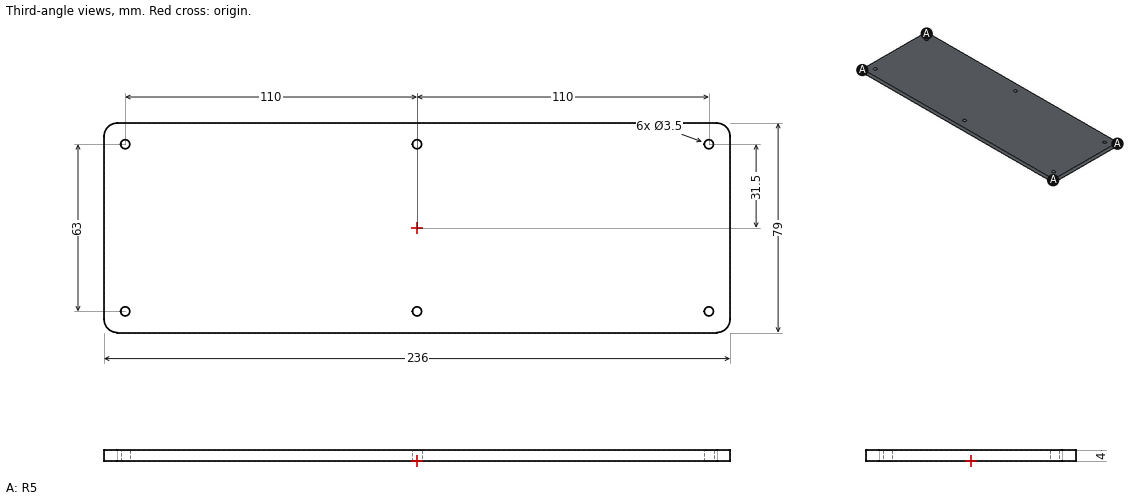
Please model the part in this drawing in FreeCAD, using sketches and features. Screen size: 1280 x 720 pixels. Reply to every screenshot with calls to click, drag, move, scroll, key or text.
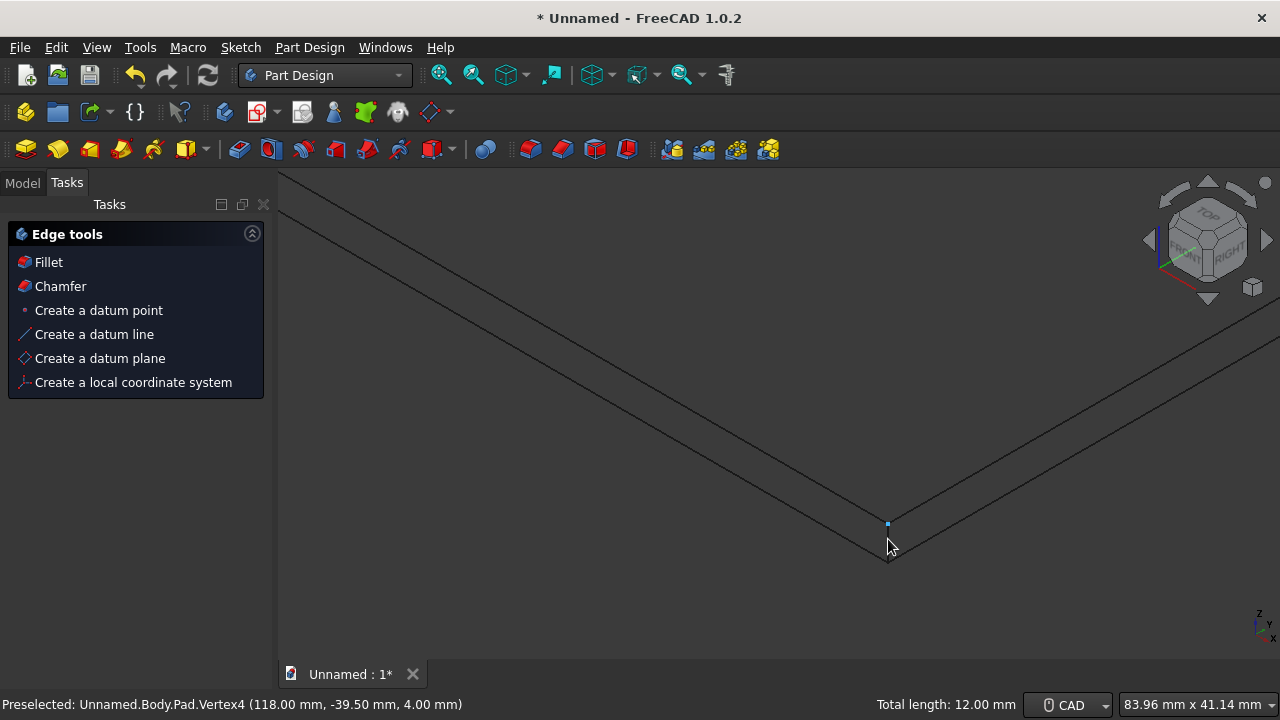
click(888, 542, ctrl)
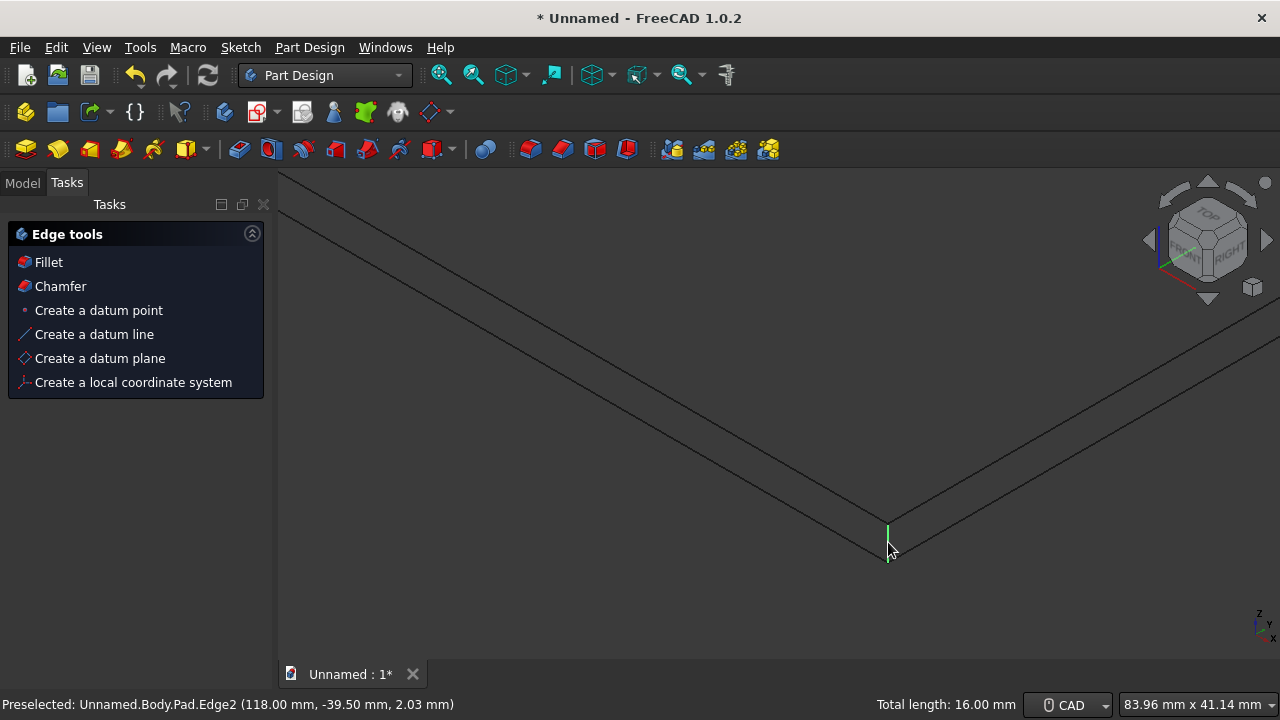
key(v)
key(1)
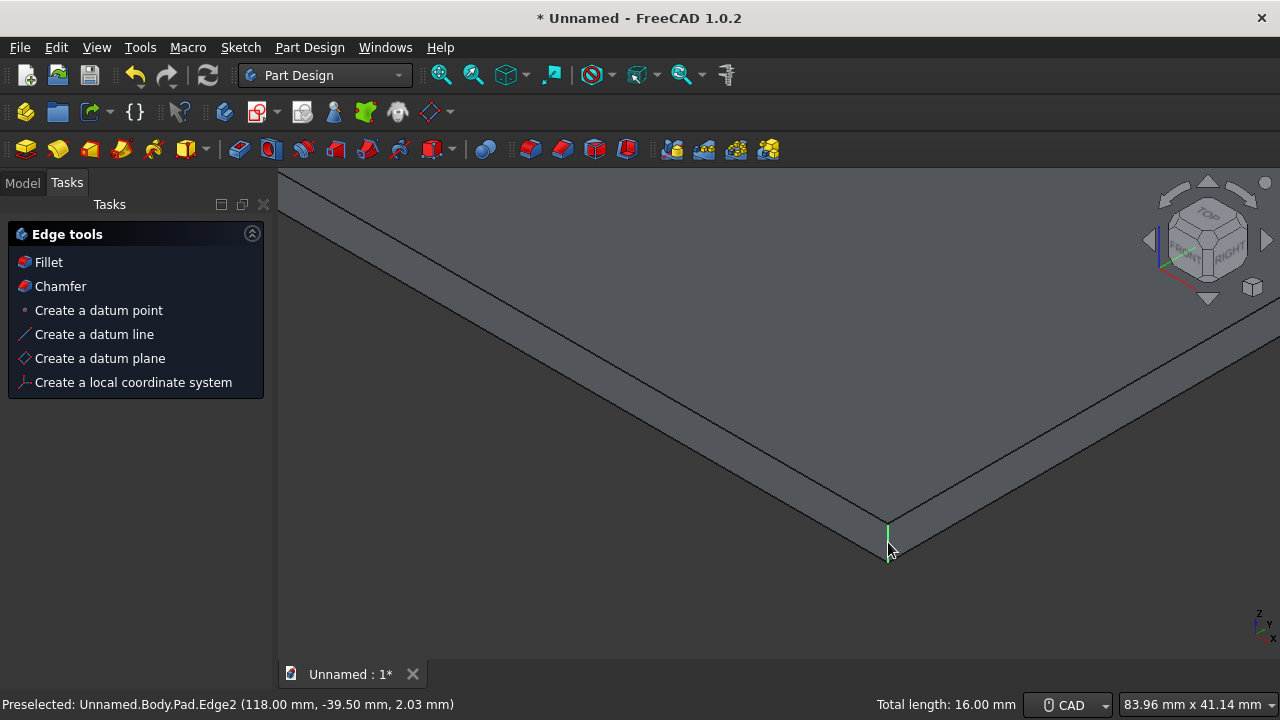
click(532, 150)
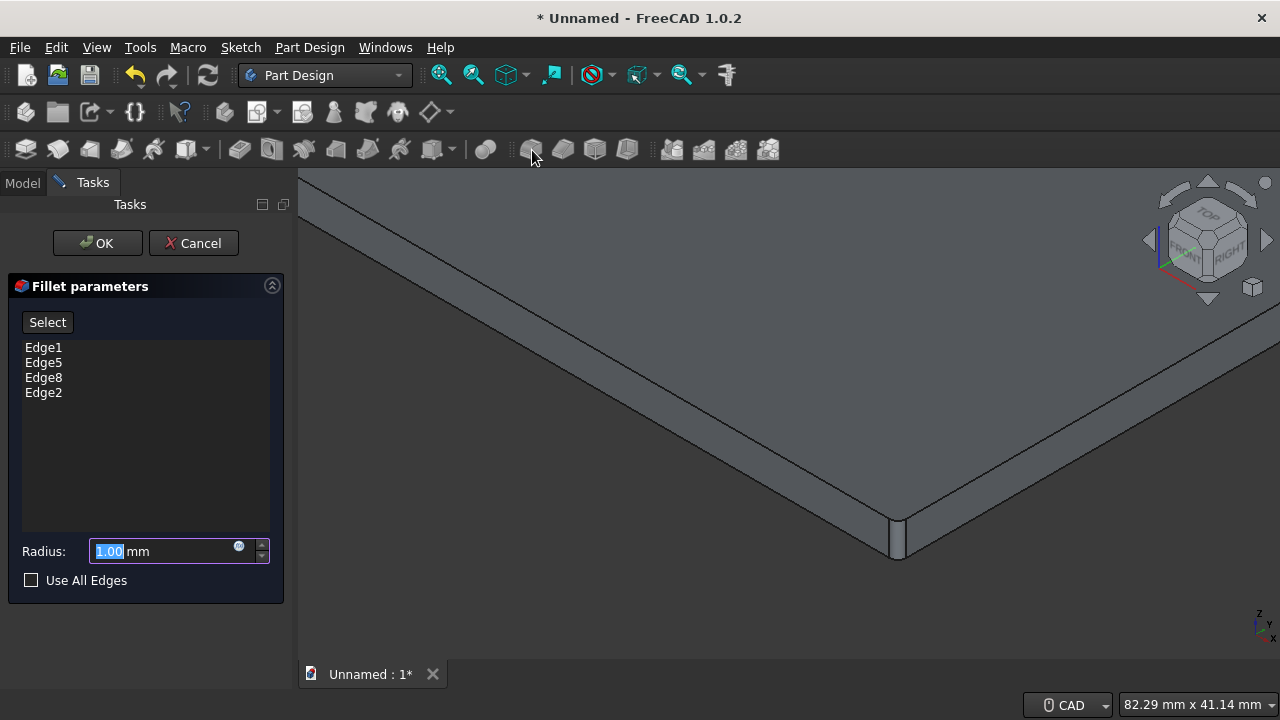
text(5)
key(Tab)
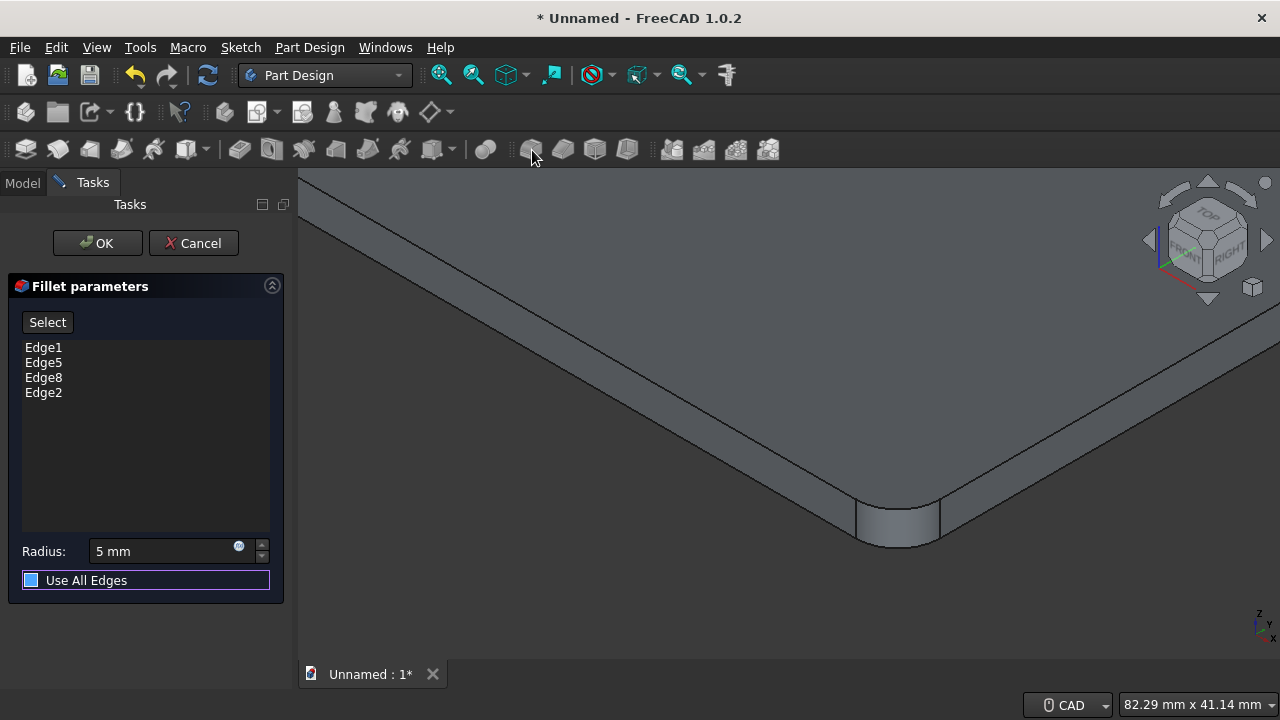
click(98, 243)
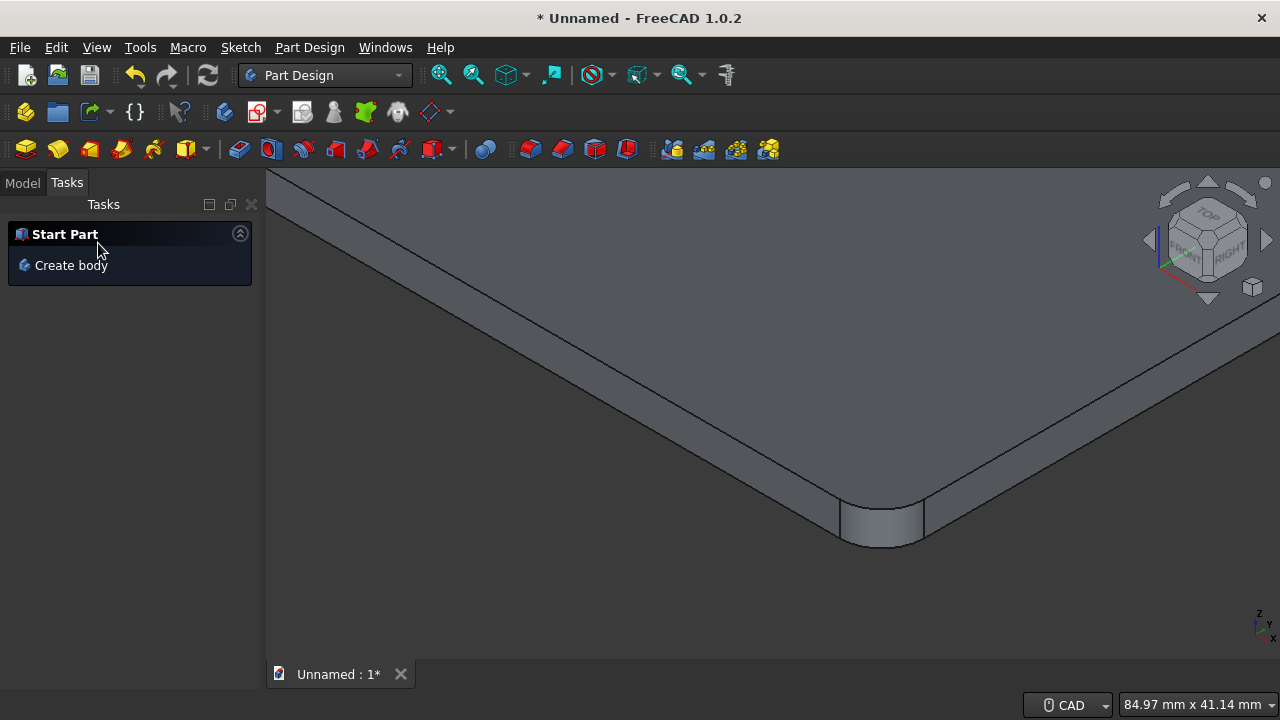
click(442, 76)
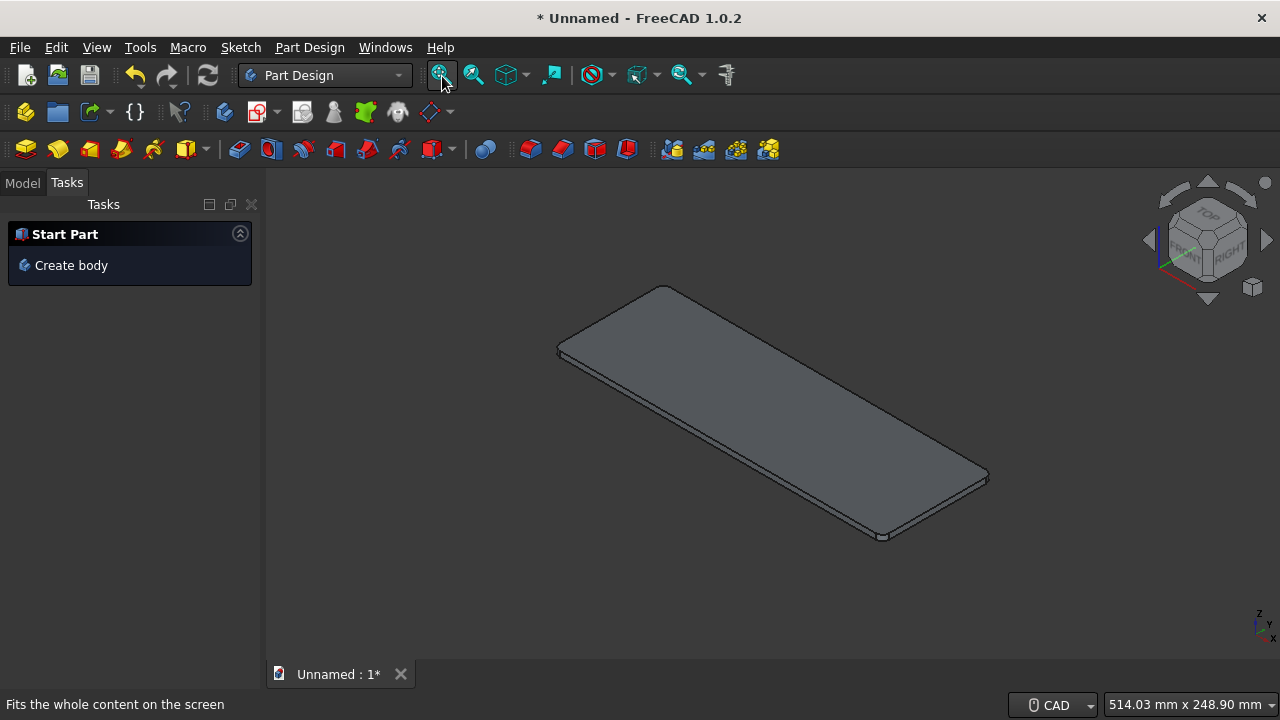
click(258, 112)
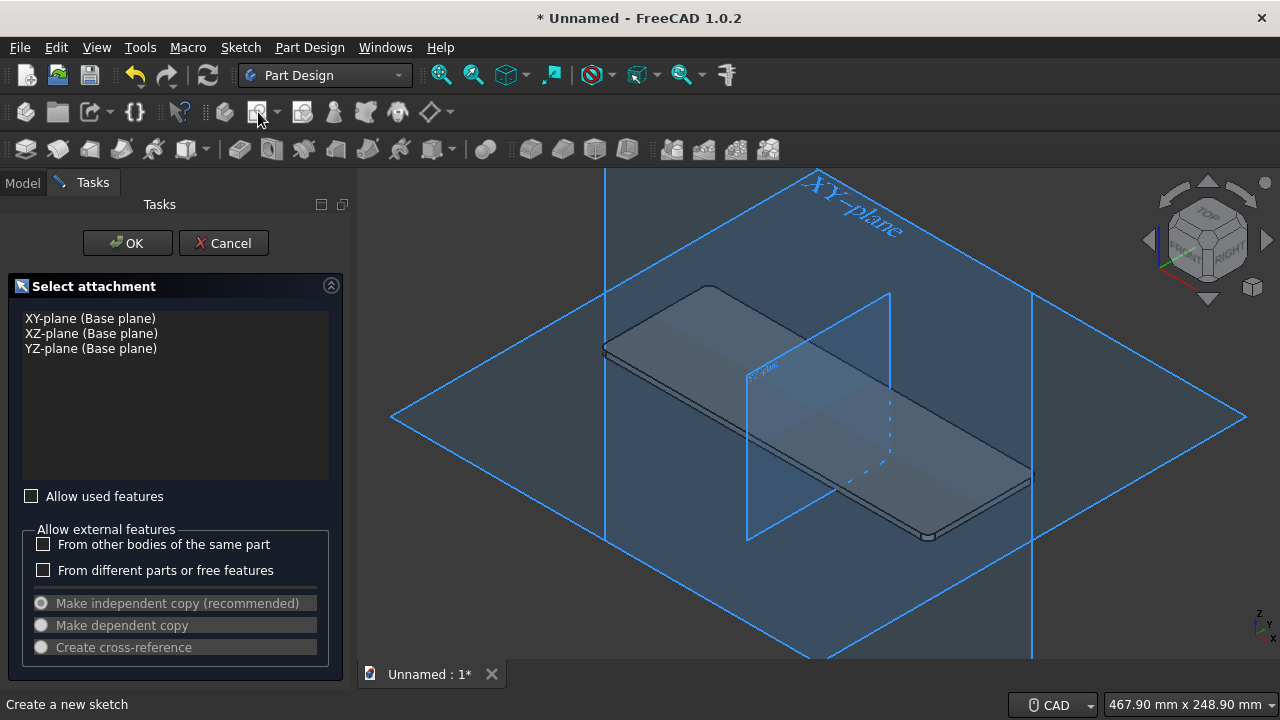
click(82, 318)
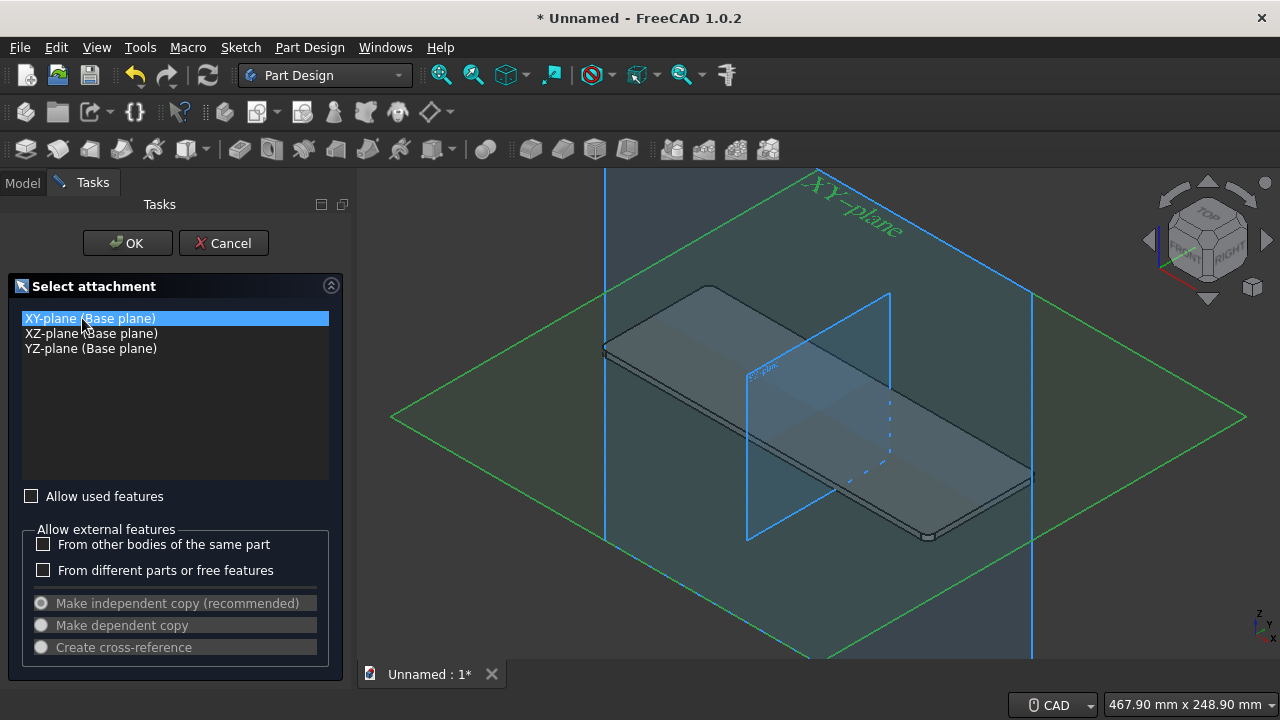
click(128, 243)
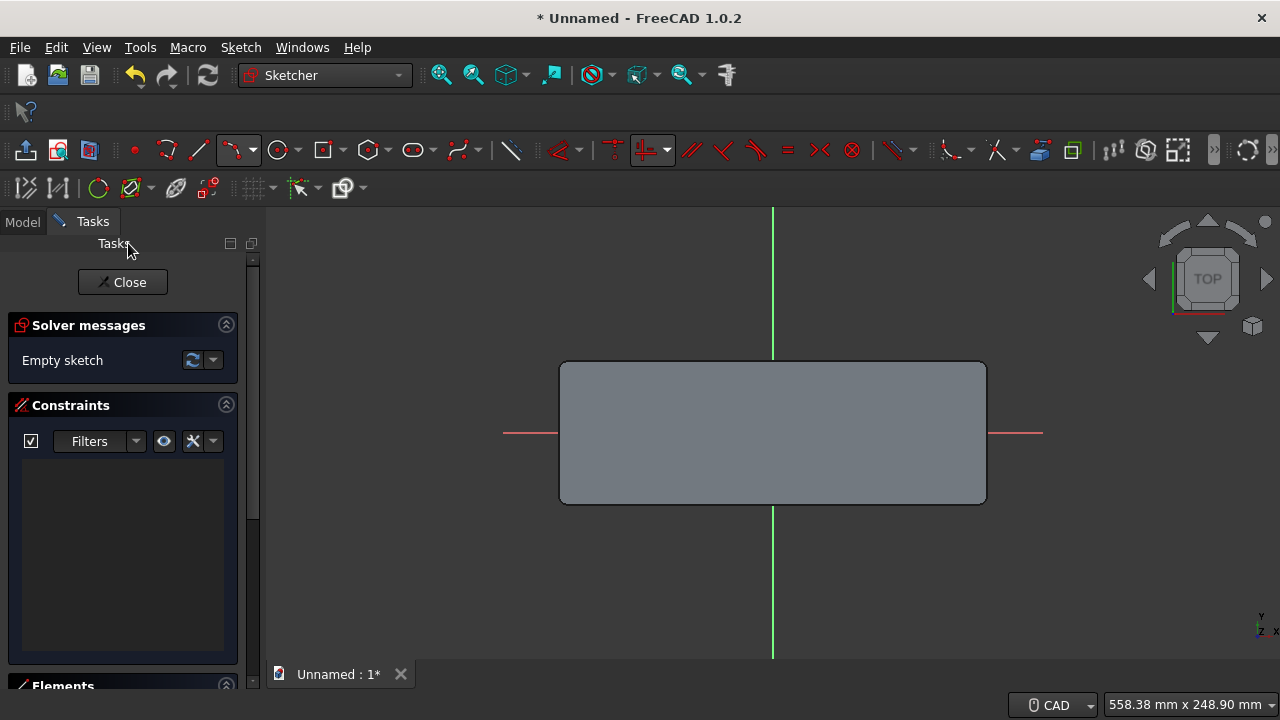
click(90, 150)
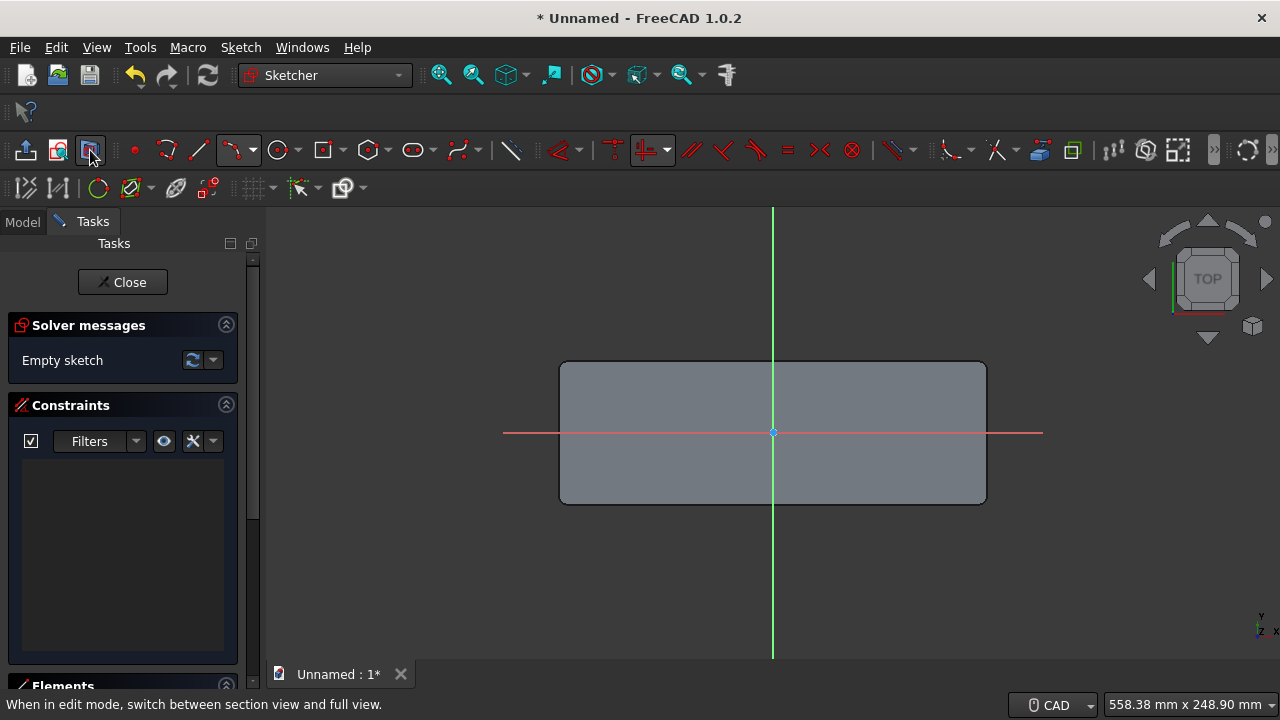
scroll(912, 433, up, 2)